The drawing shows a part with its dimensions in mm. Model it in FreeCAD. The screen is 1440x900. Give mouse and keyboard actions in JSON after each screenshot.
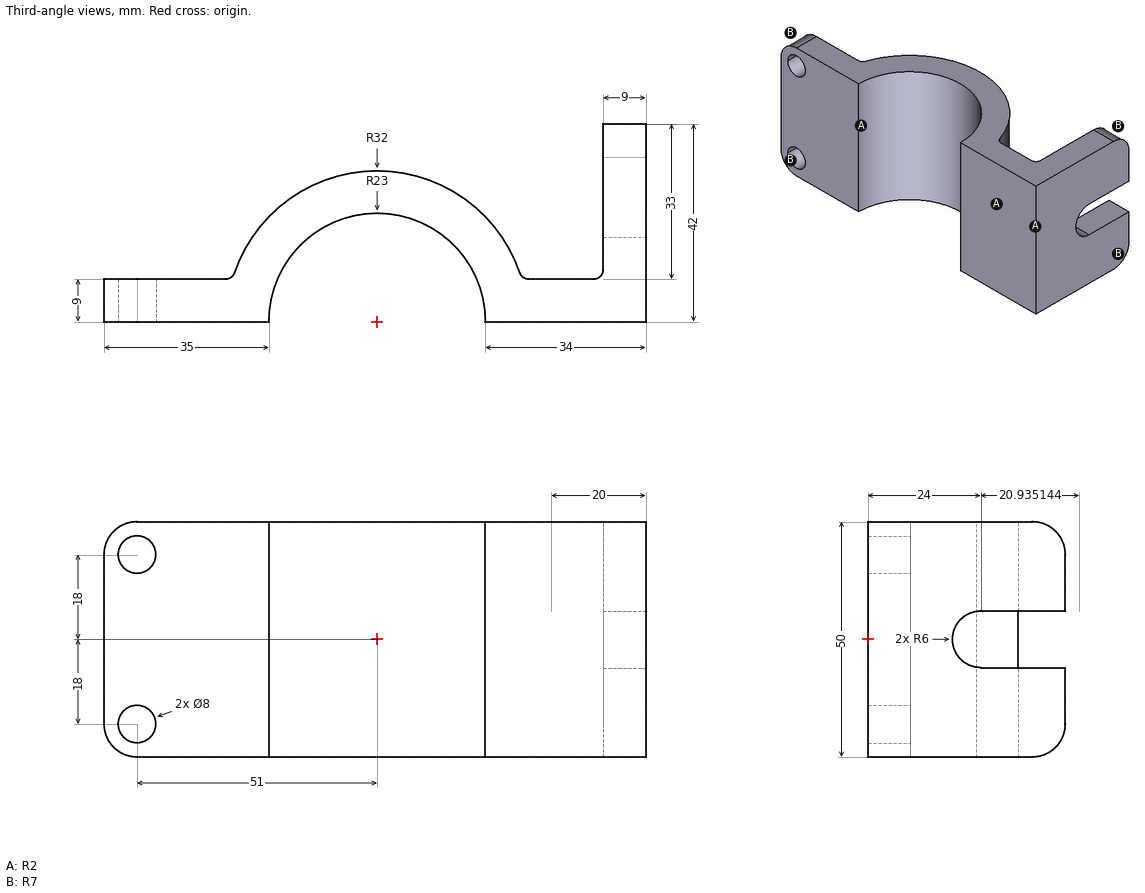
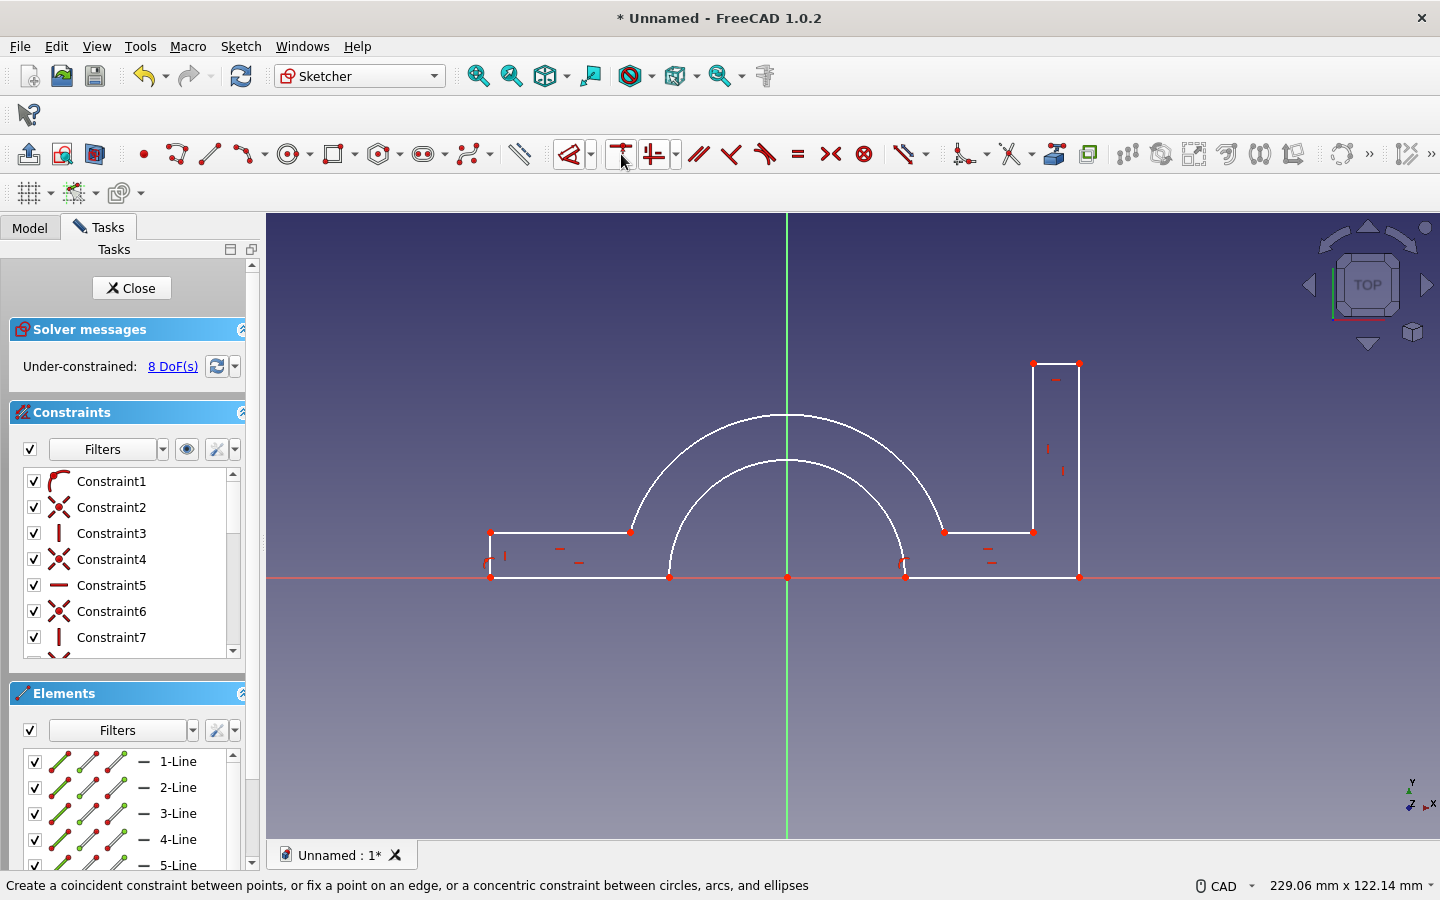
{"action": "left_click", "coordinate": [568, 154]}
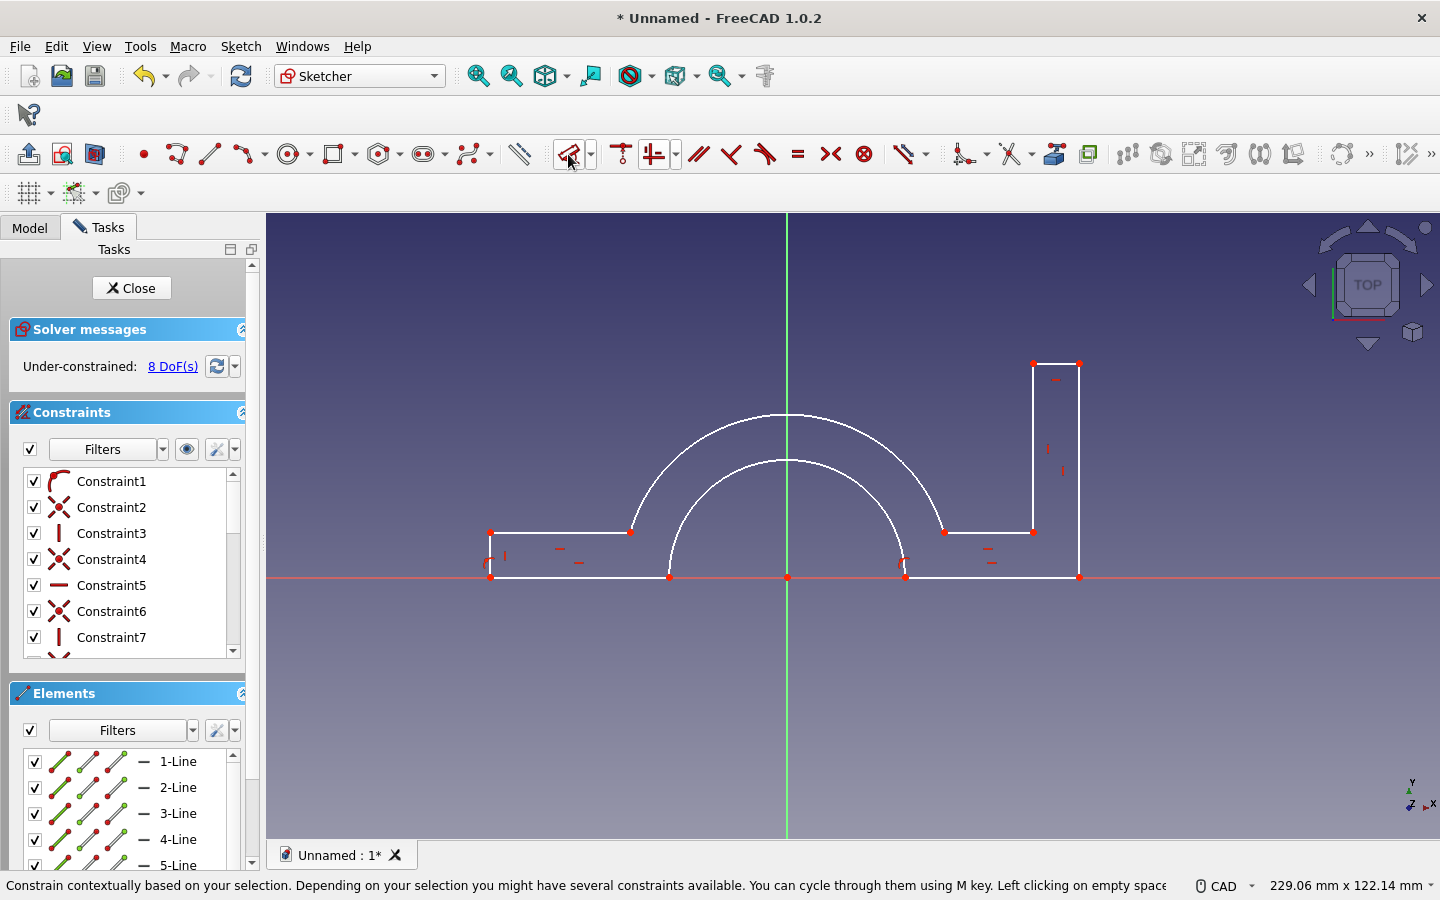
{"action": "left_click", "coordinate": [868, 436]}
{"action": "left_click", "coordinate": [884, 408]}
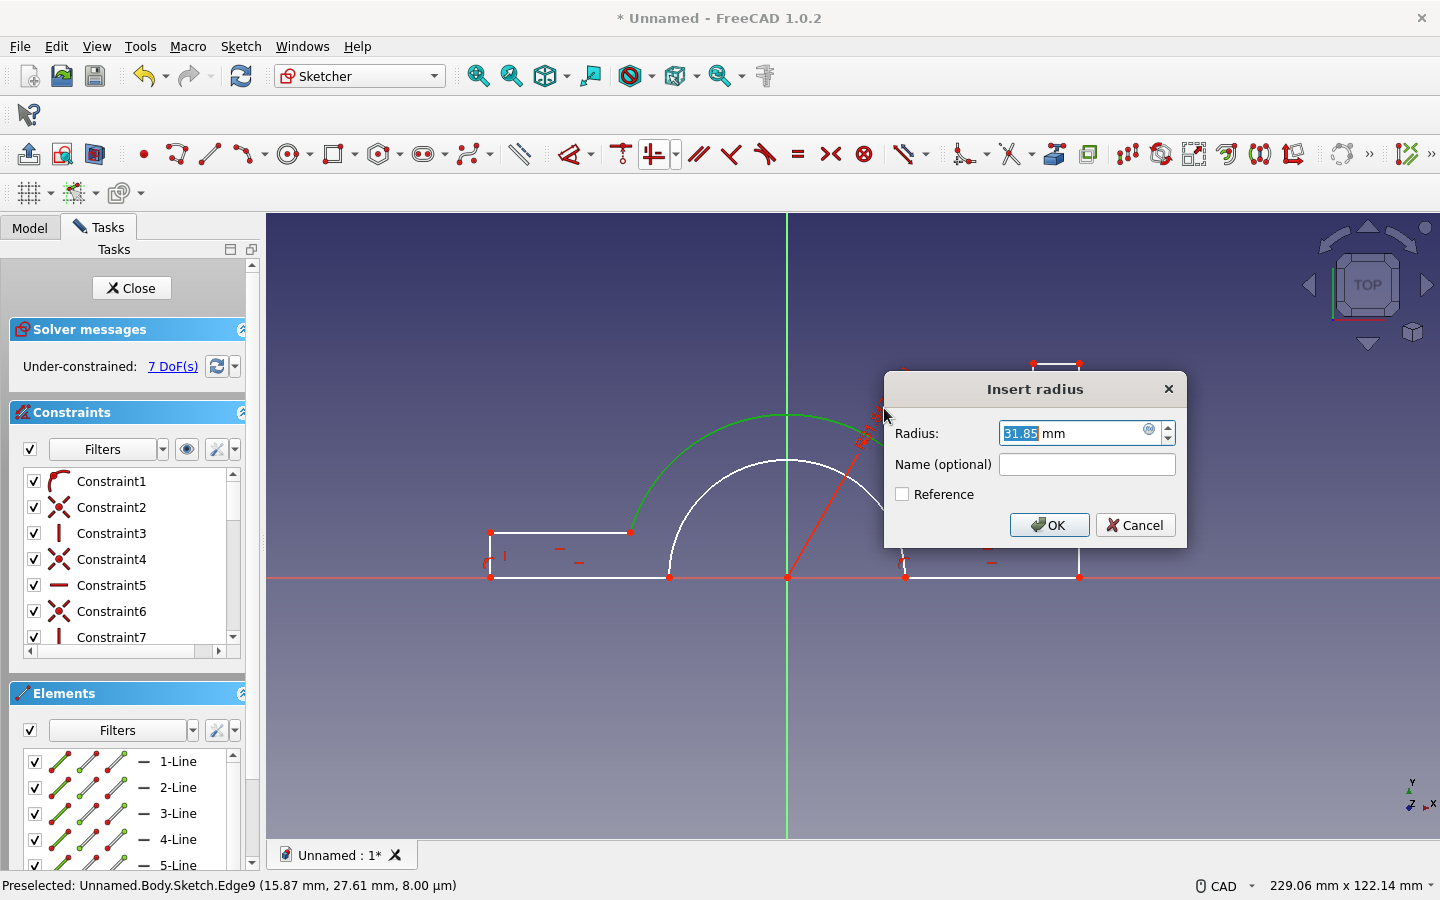
{"action": "type", "text": "32"}
{"action": "key", "text": "Return"}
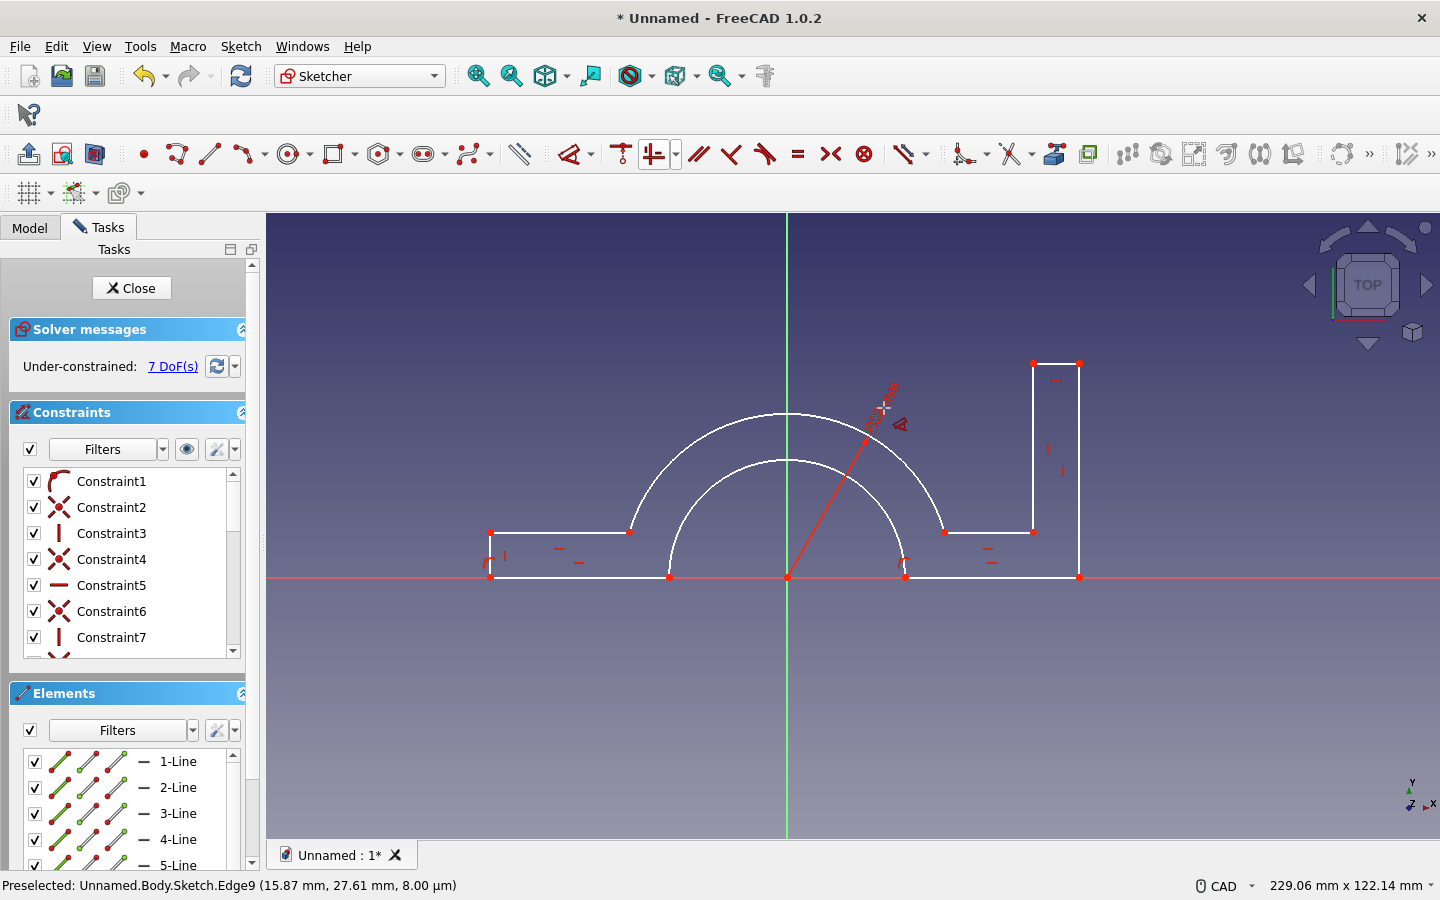
{"action": "left_click", "coordinate": [856, 482]}
{"action": "left_click", "coordinate": [875, 456]}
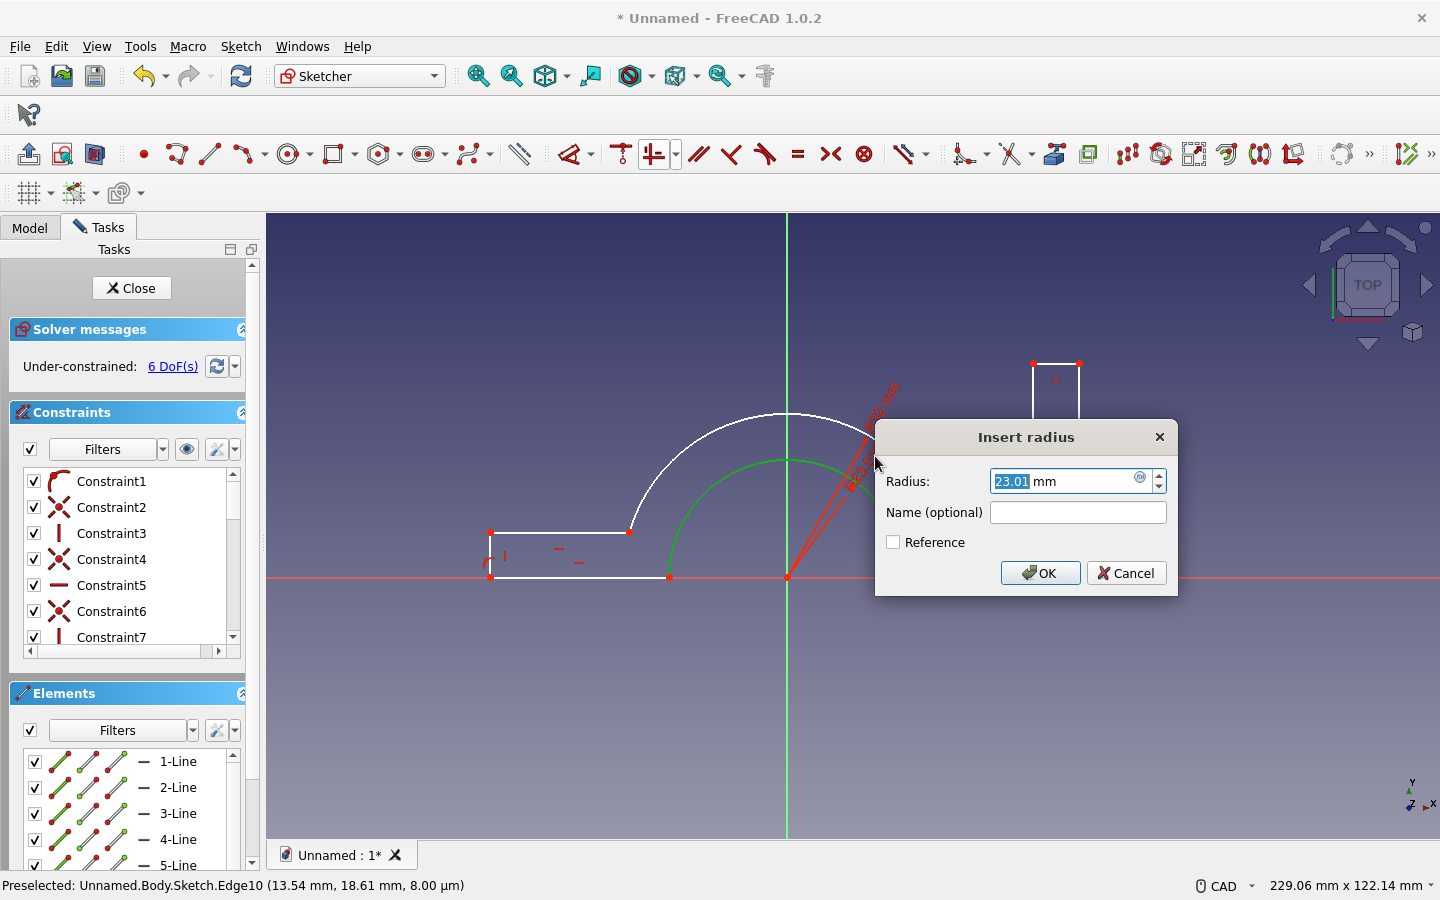
{"action": "type", "text": "23"}
{"action": "key", "text": "Return"}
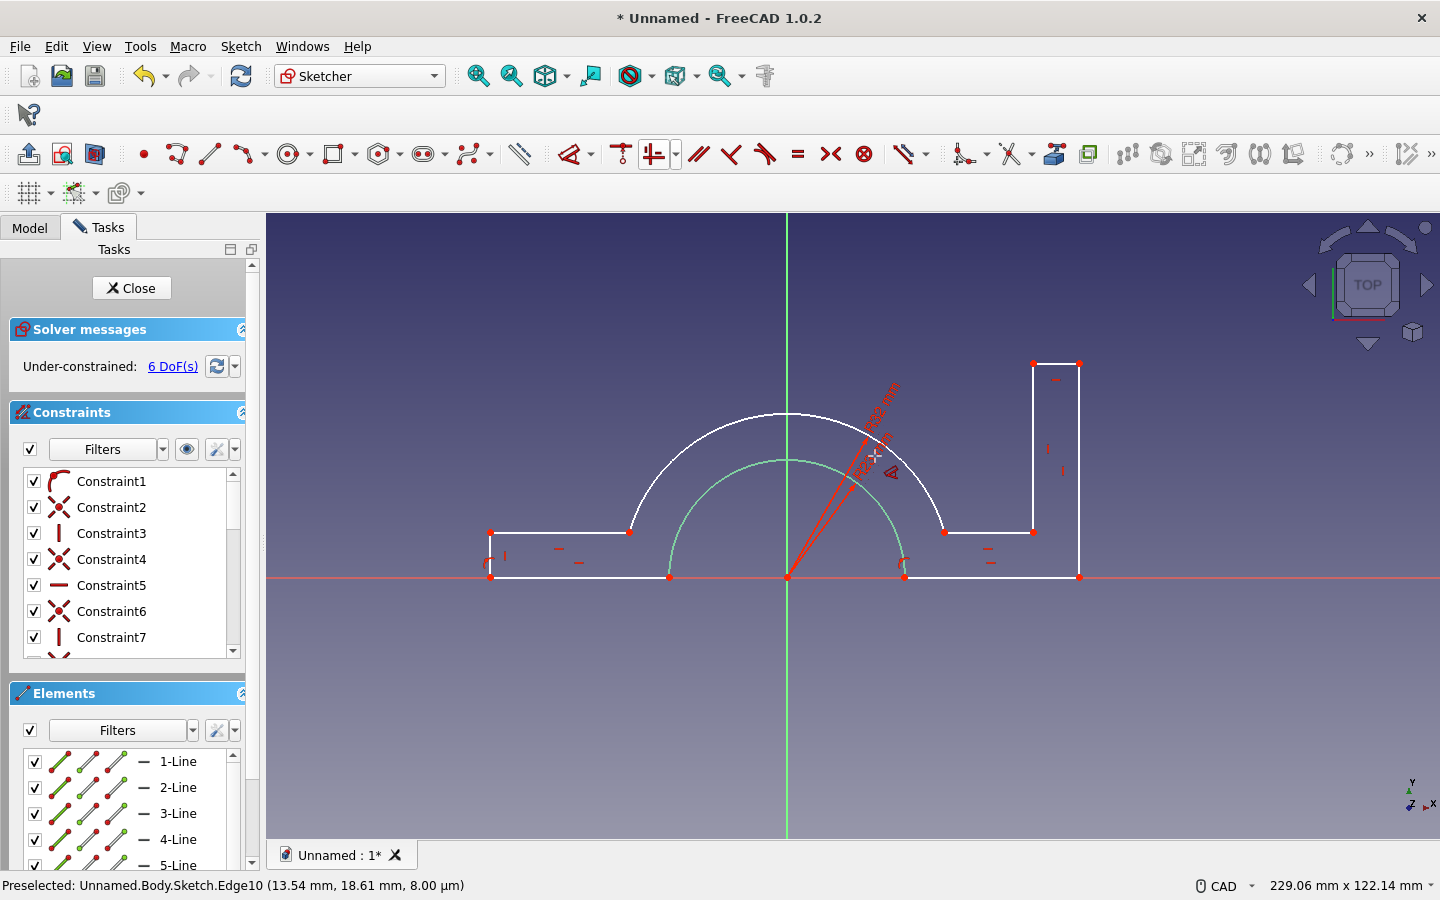
{"action": "left_click", "coordinate": [1065, 364]}
{"action": "left_click", "coordinate": [1056, 330]}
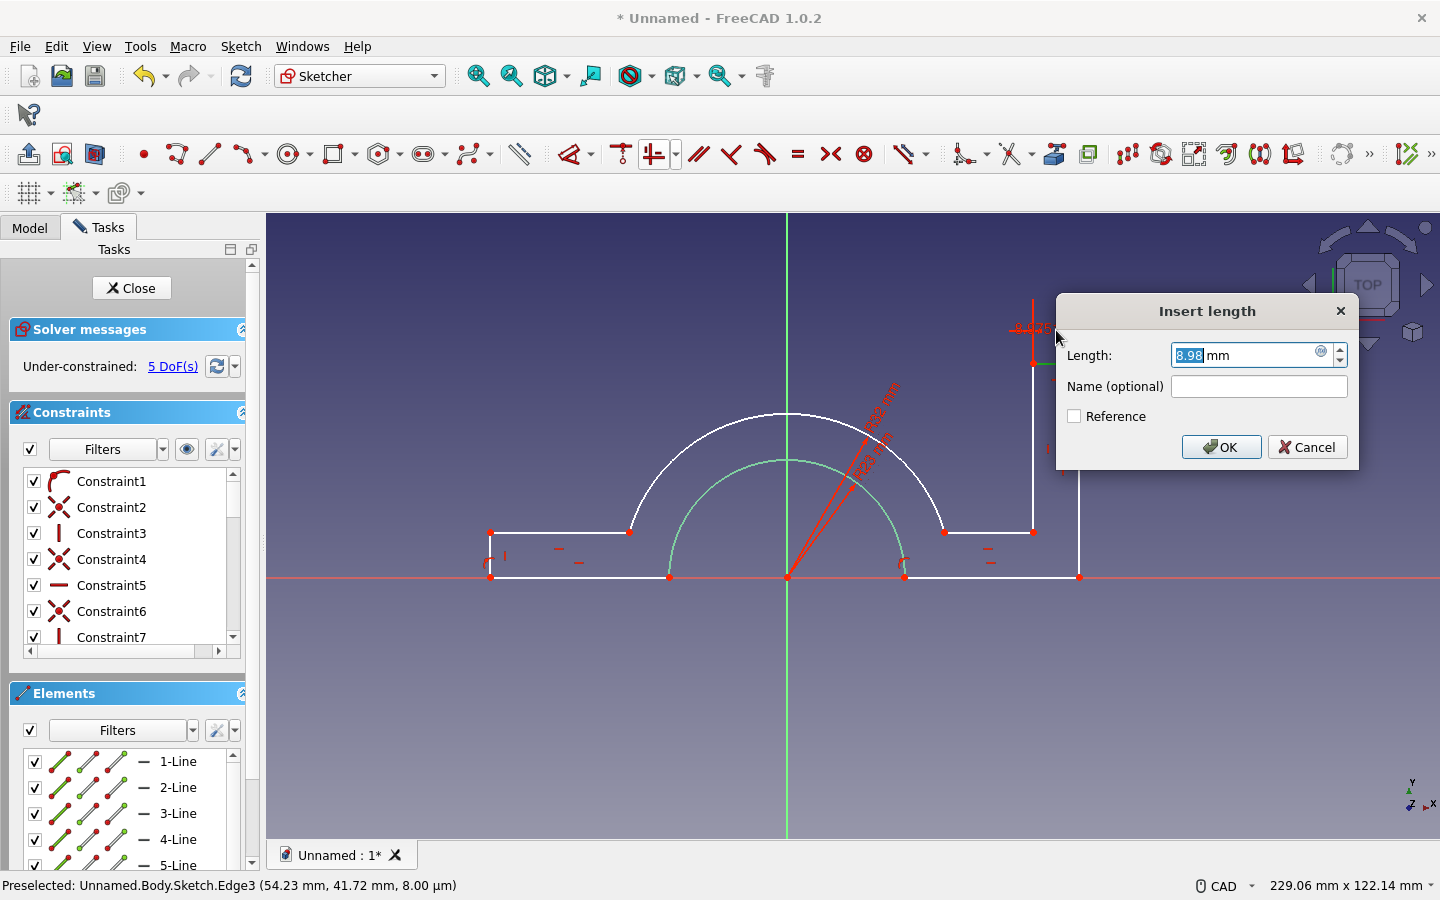
{"action": "type", "text": "9"}
{"action": "key", "text": "Return"}